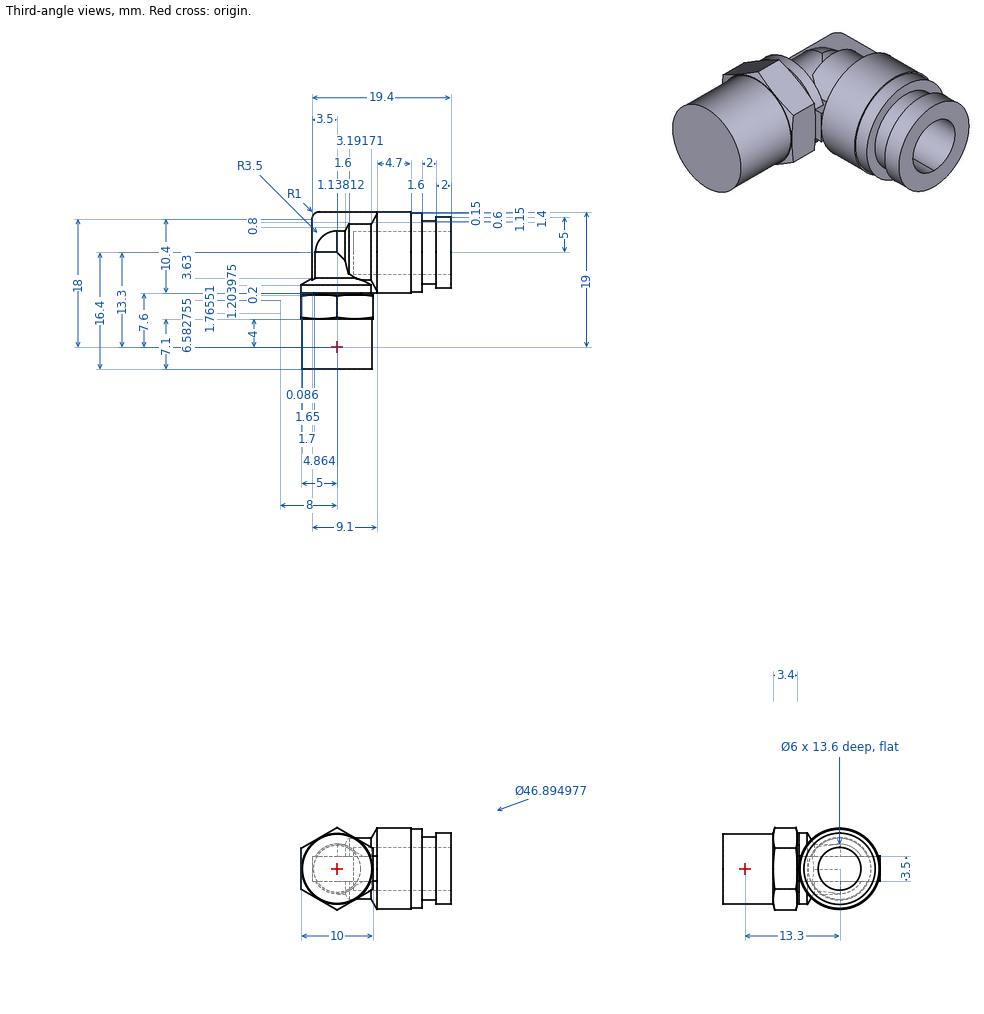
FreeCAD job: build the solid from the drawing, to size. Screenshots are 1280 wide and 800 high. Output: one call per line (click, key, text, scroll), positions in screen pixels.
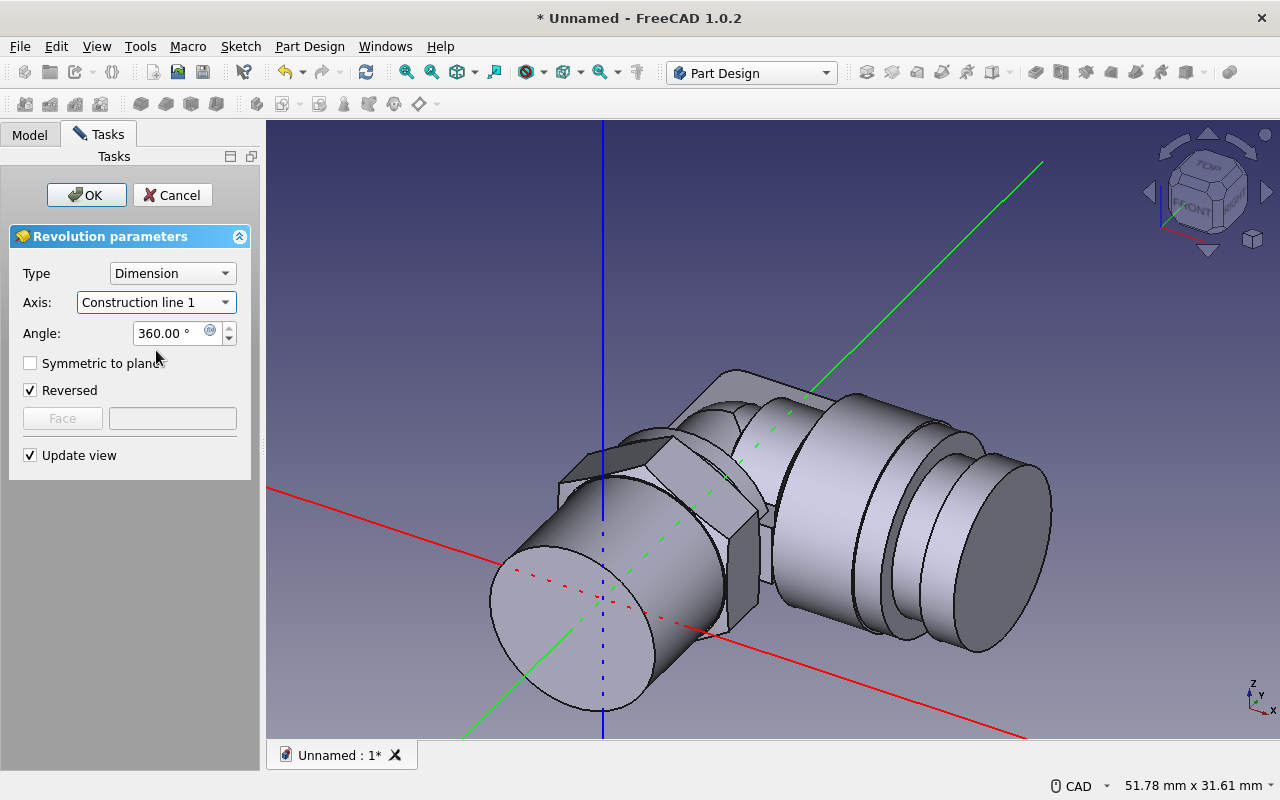
click(87, 195)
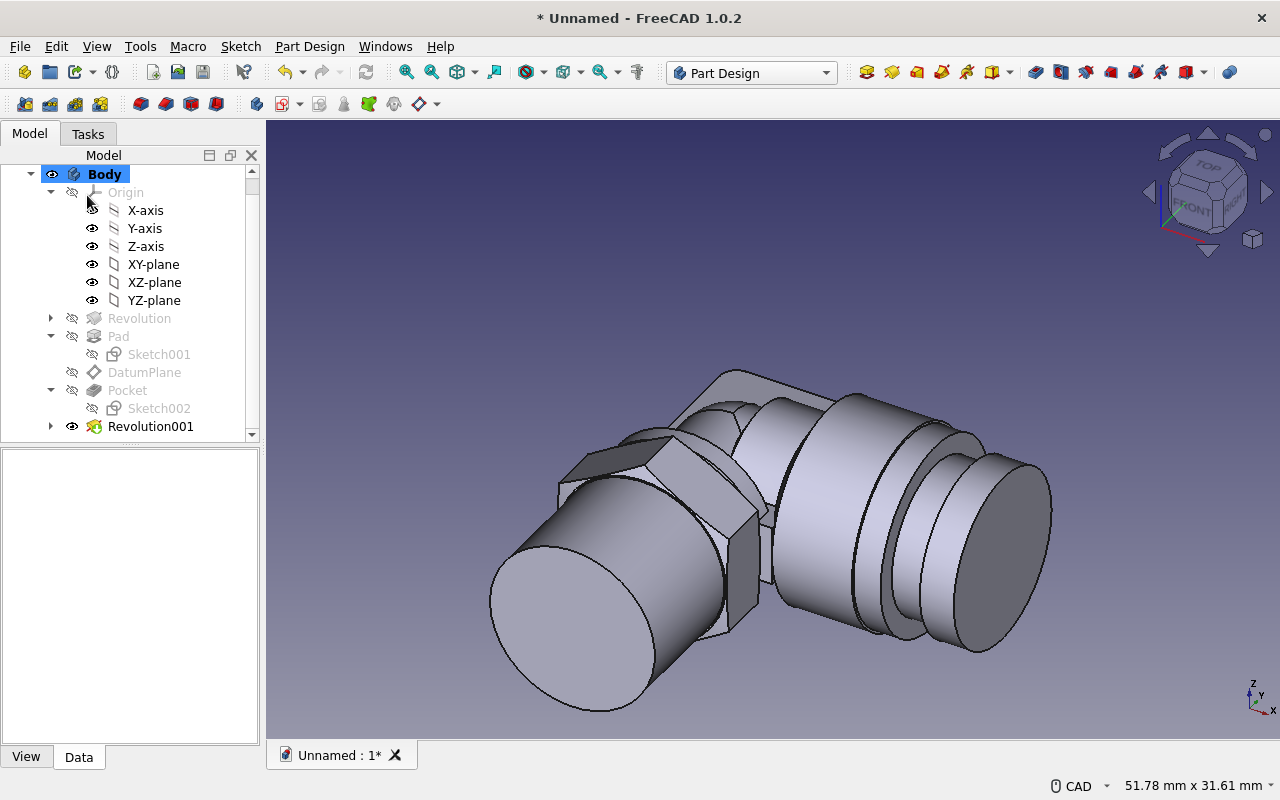
click(407, 72)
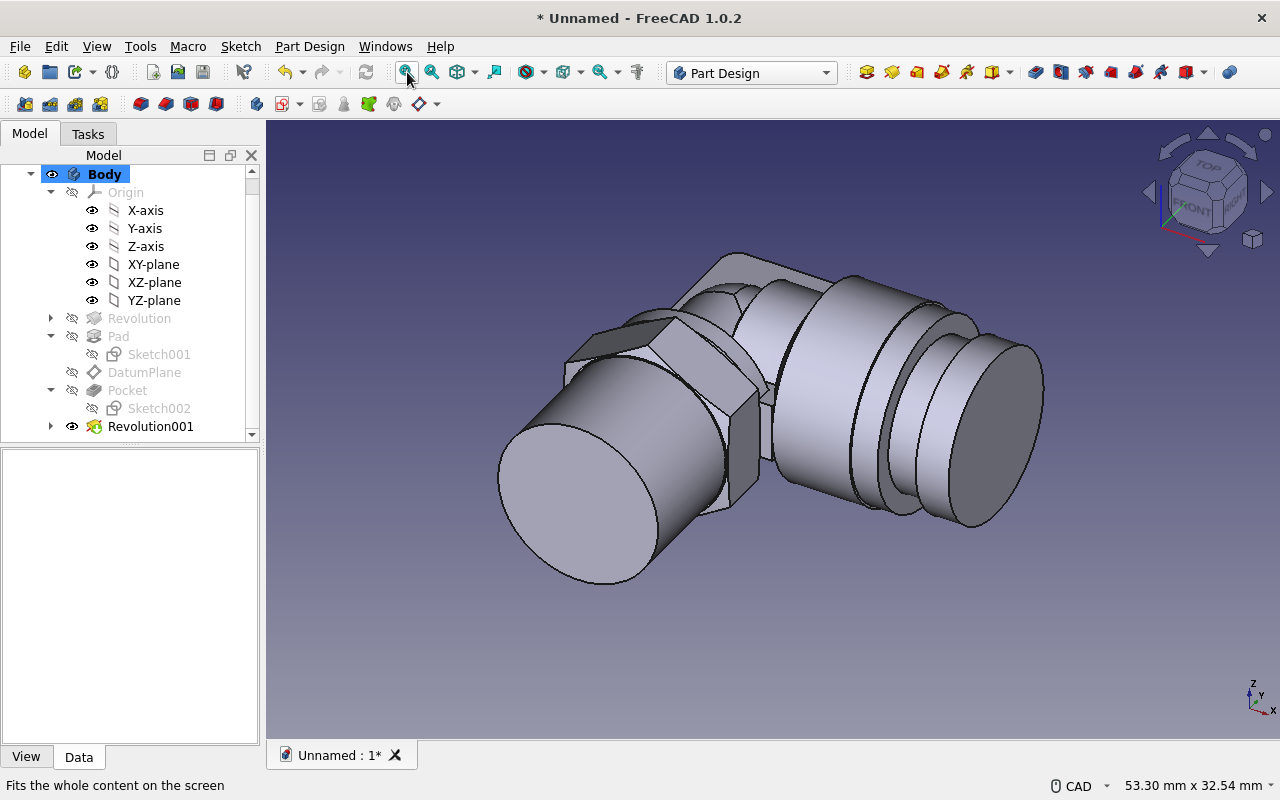
click(996, 435)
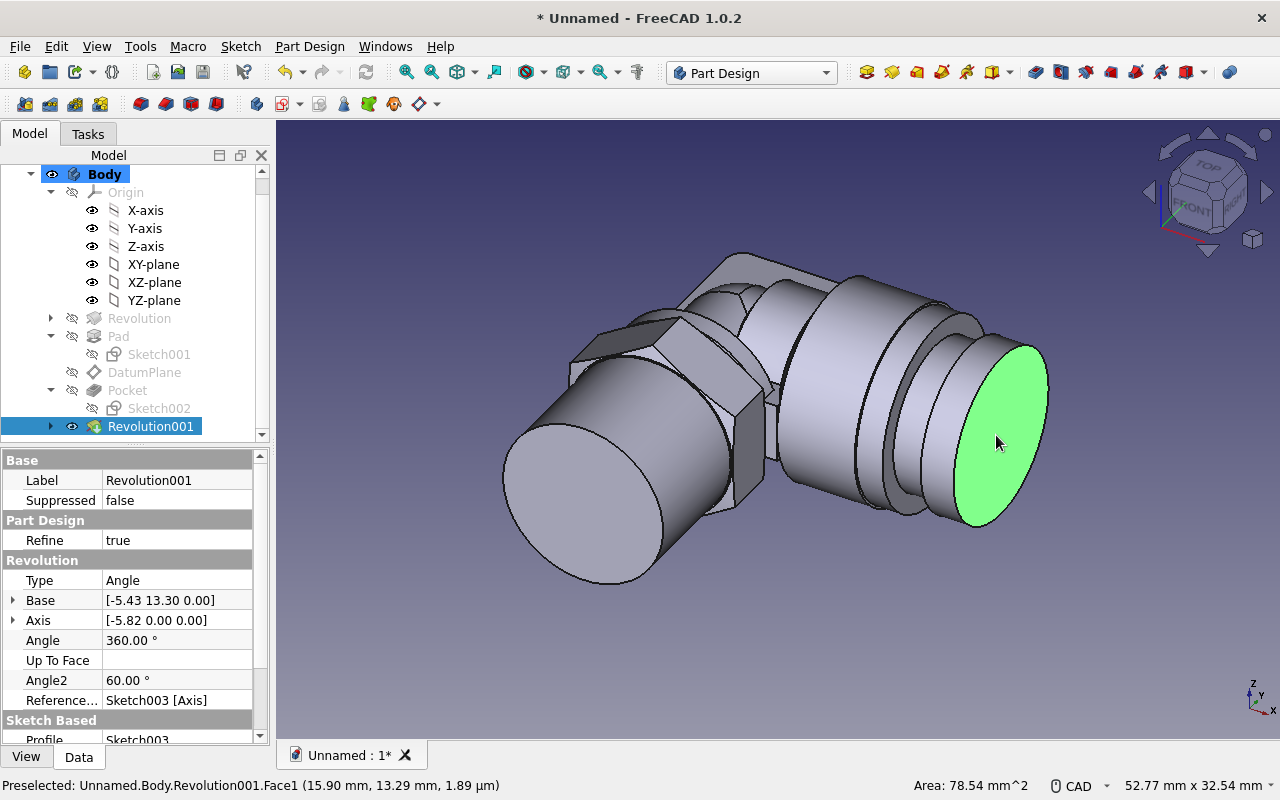
click(282, 104)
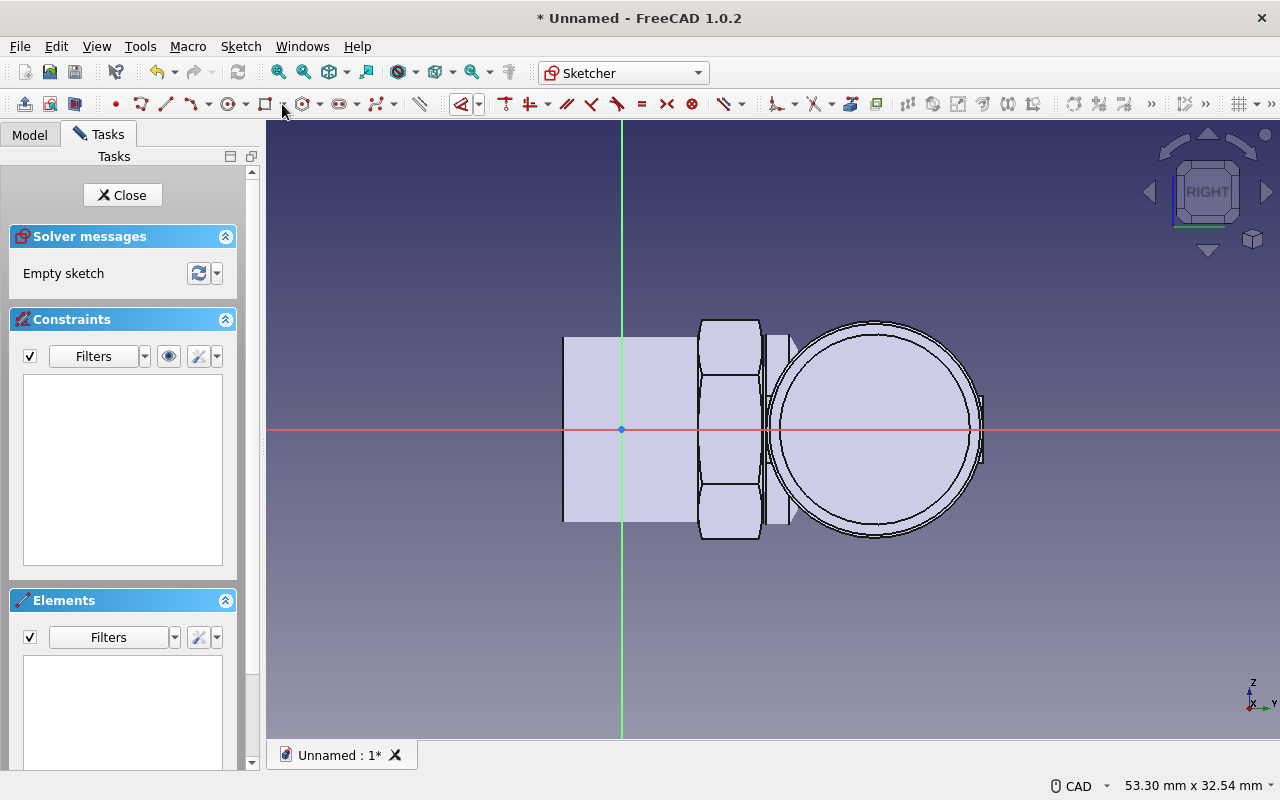
scroll(948, 430, up, 6)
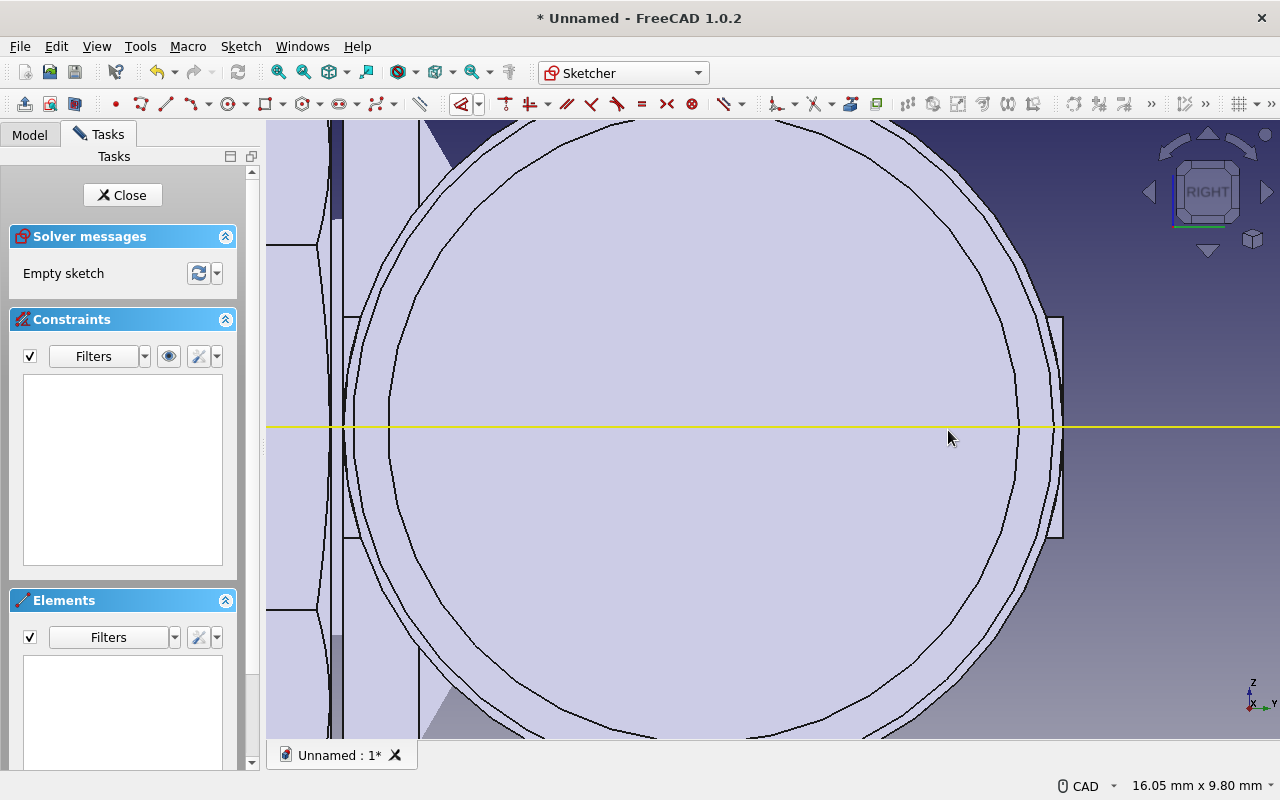
key(g)
key(c)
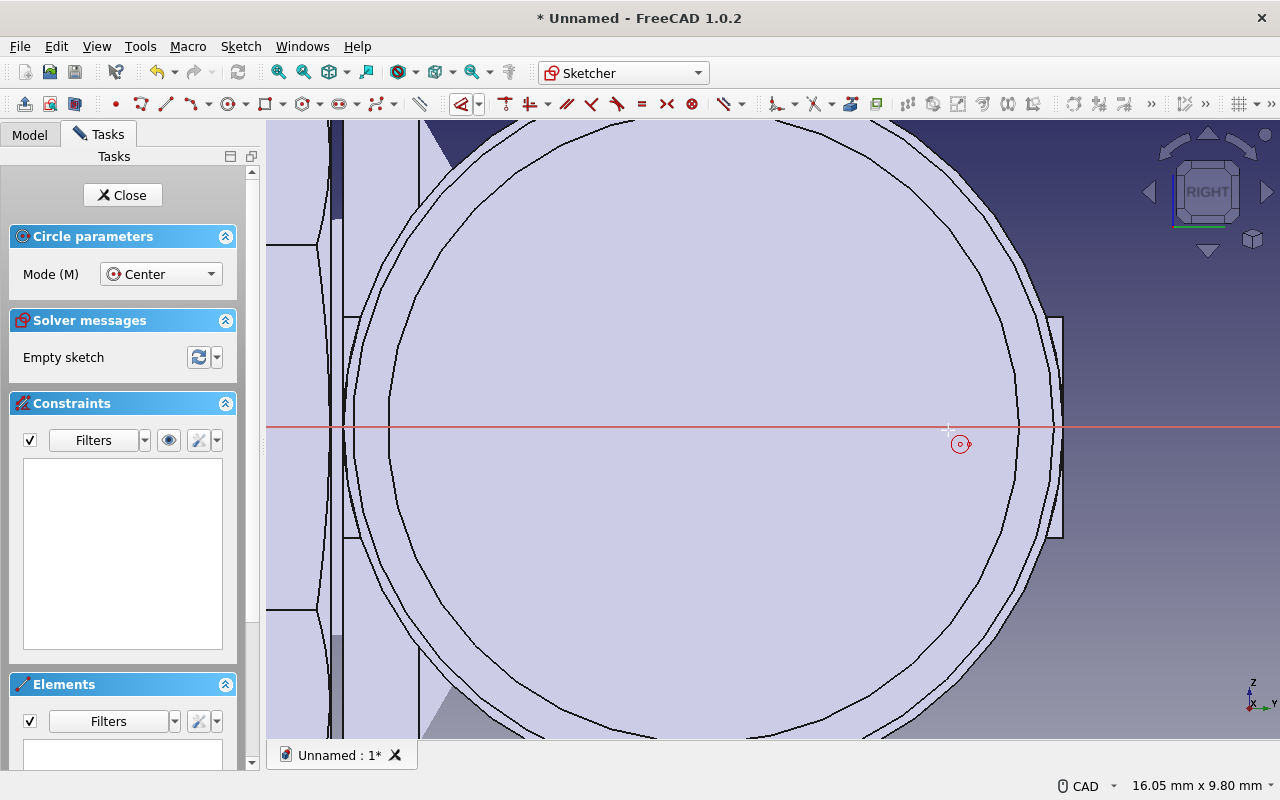
click(703, 427)
click(837, 293)
key(Escape)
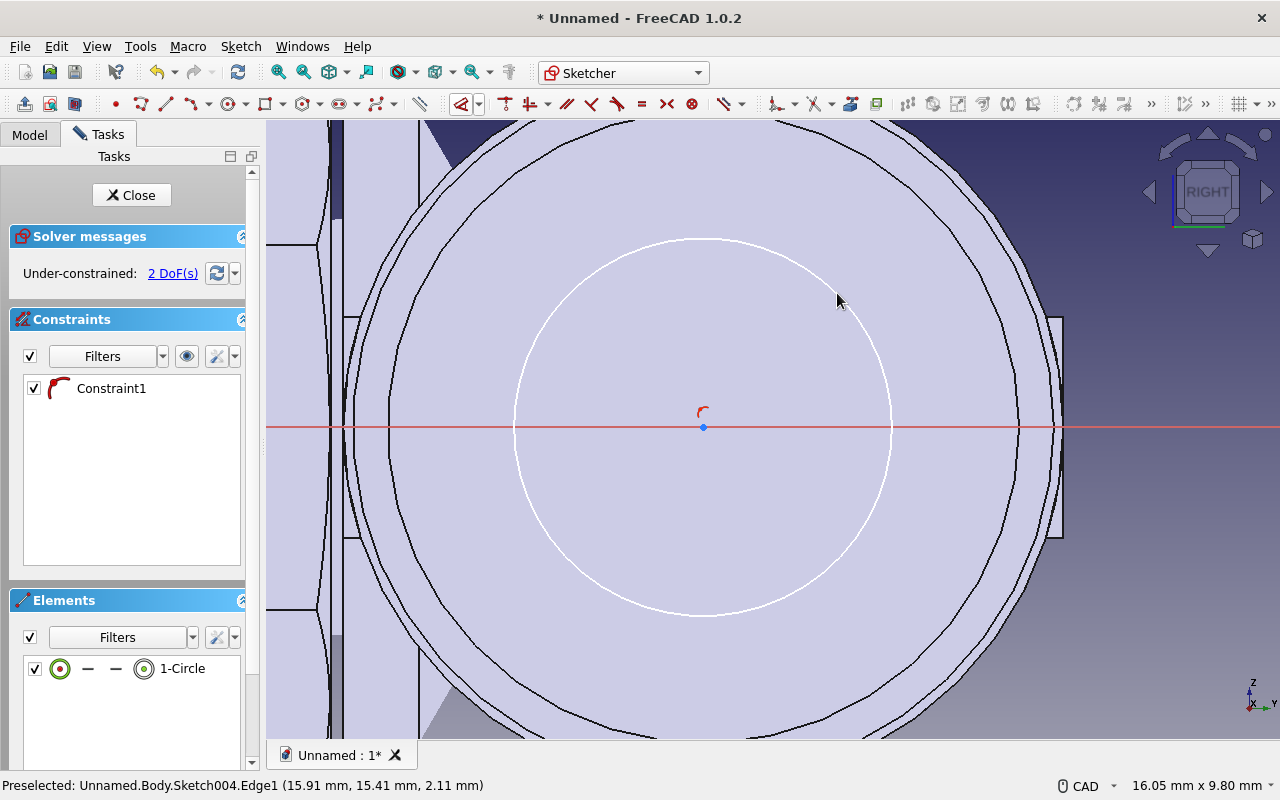
click(836, 293)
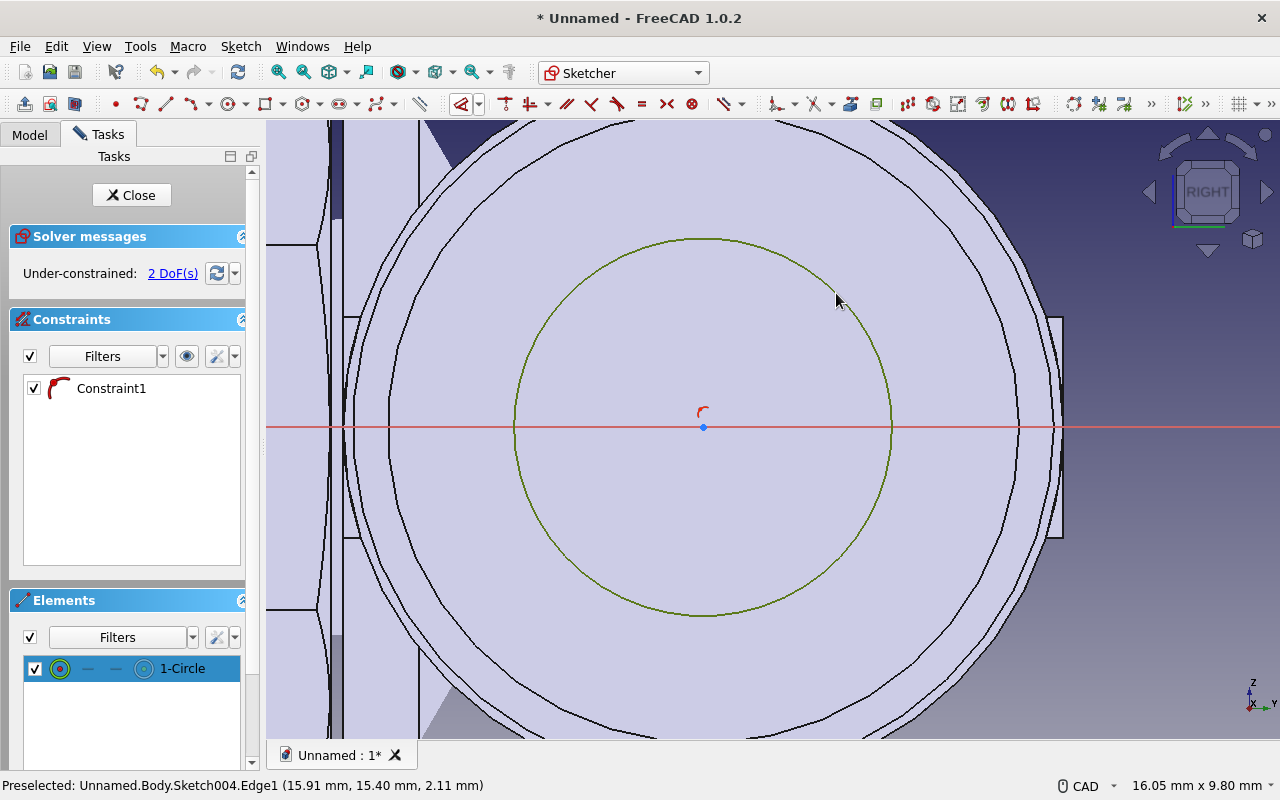
key(k)
key(o)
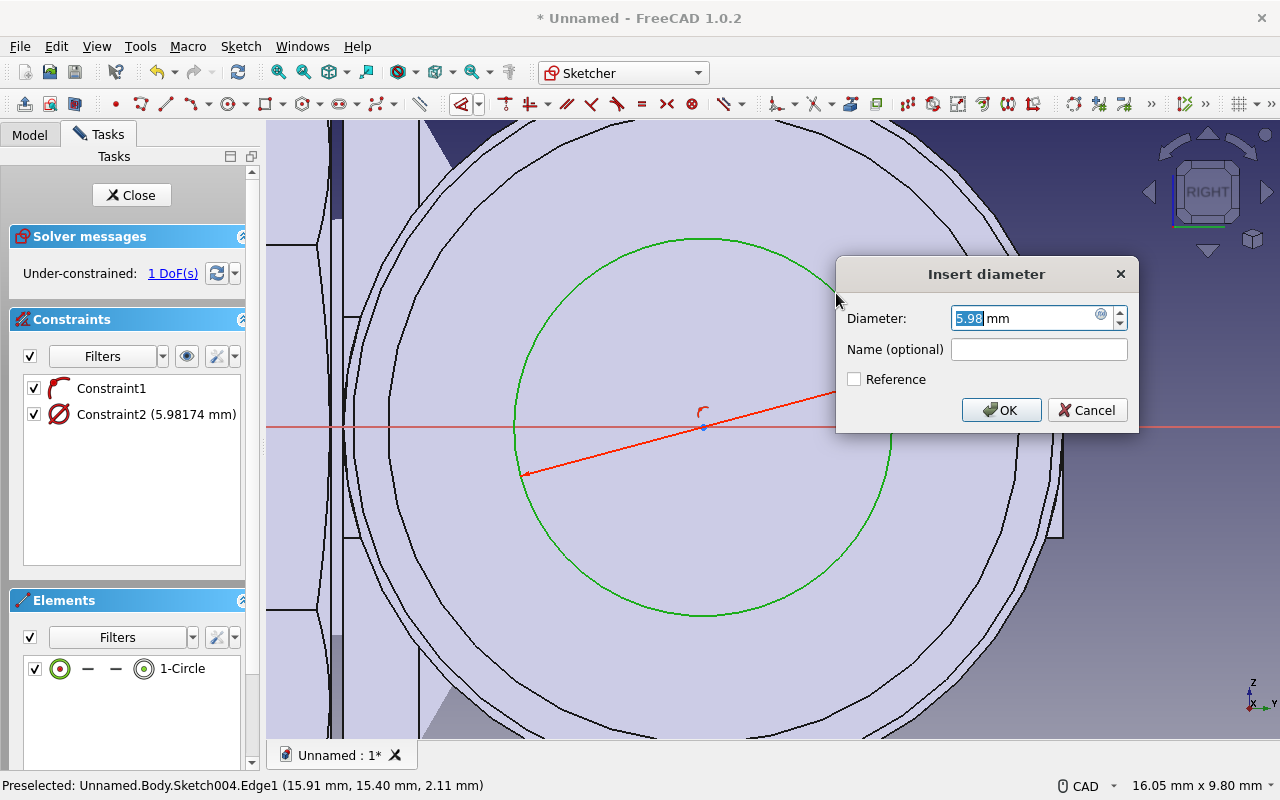
text(6)
key(Return)